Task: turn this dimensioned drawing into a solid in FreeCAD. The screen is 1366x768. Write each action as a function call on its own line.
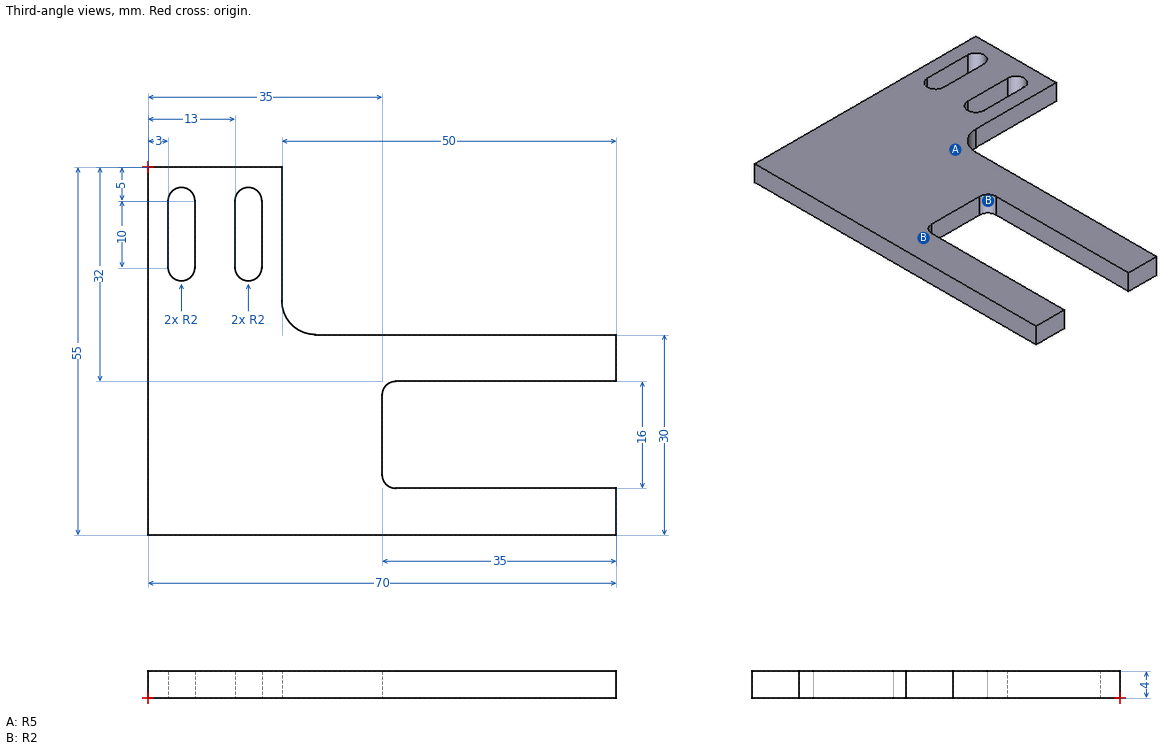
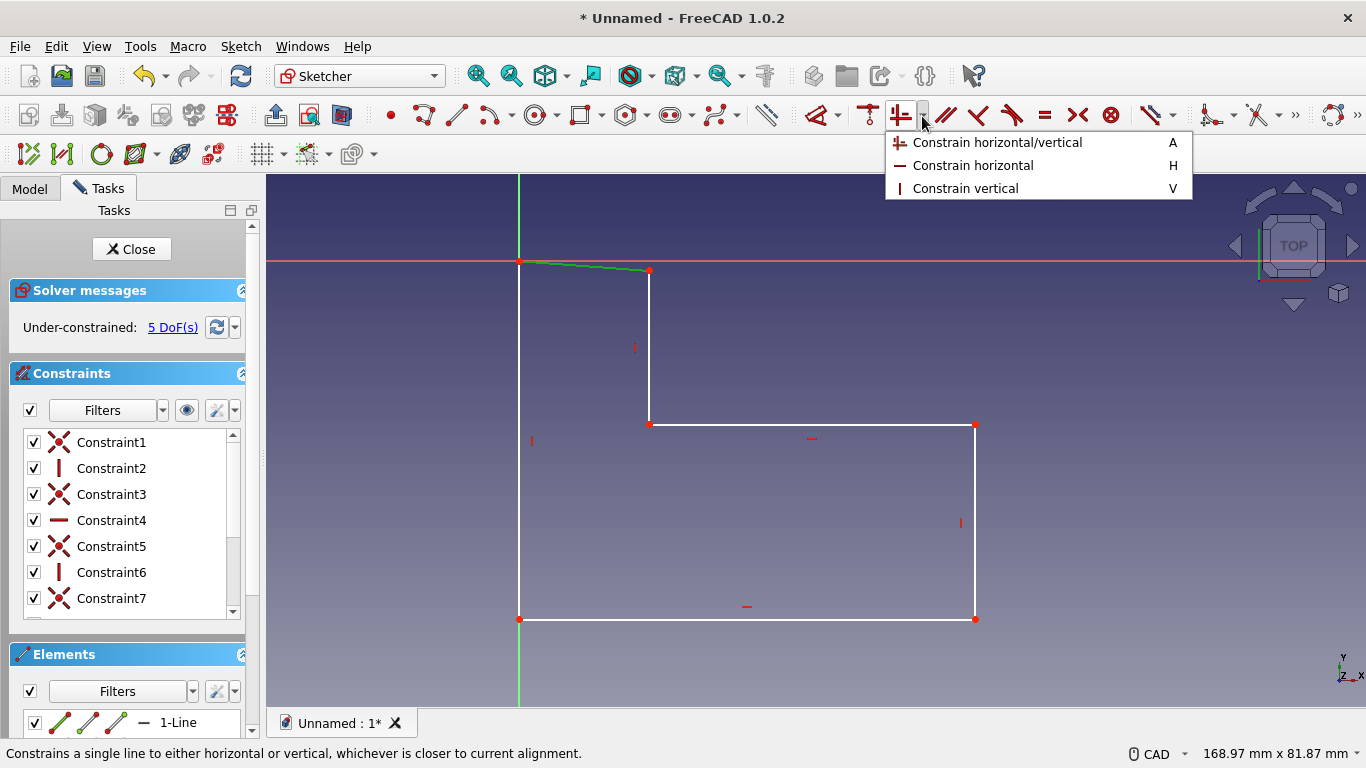
click(1039, 166)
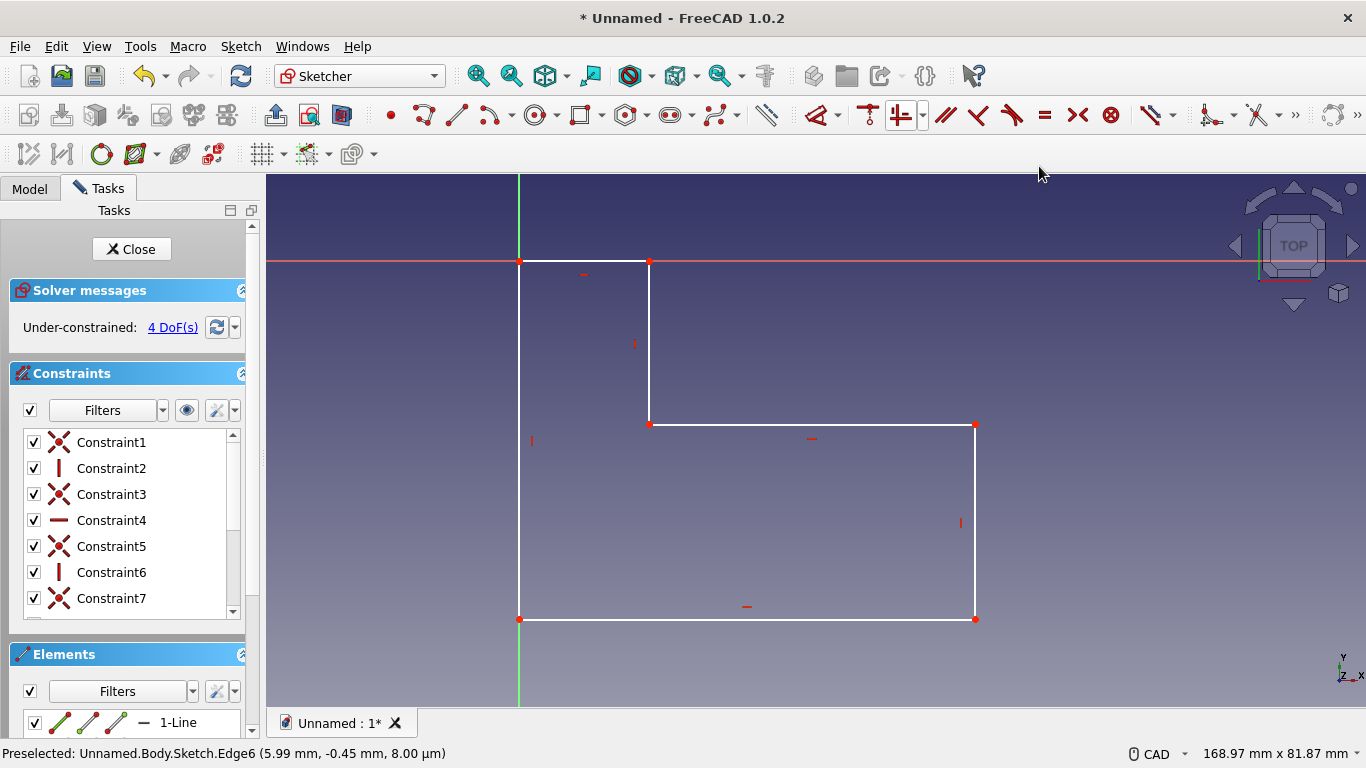
click(816, 116)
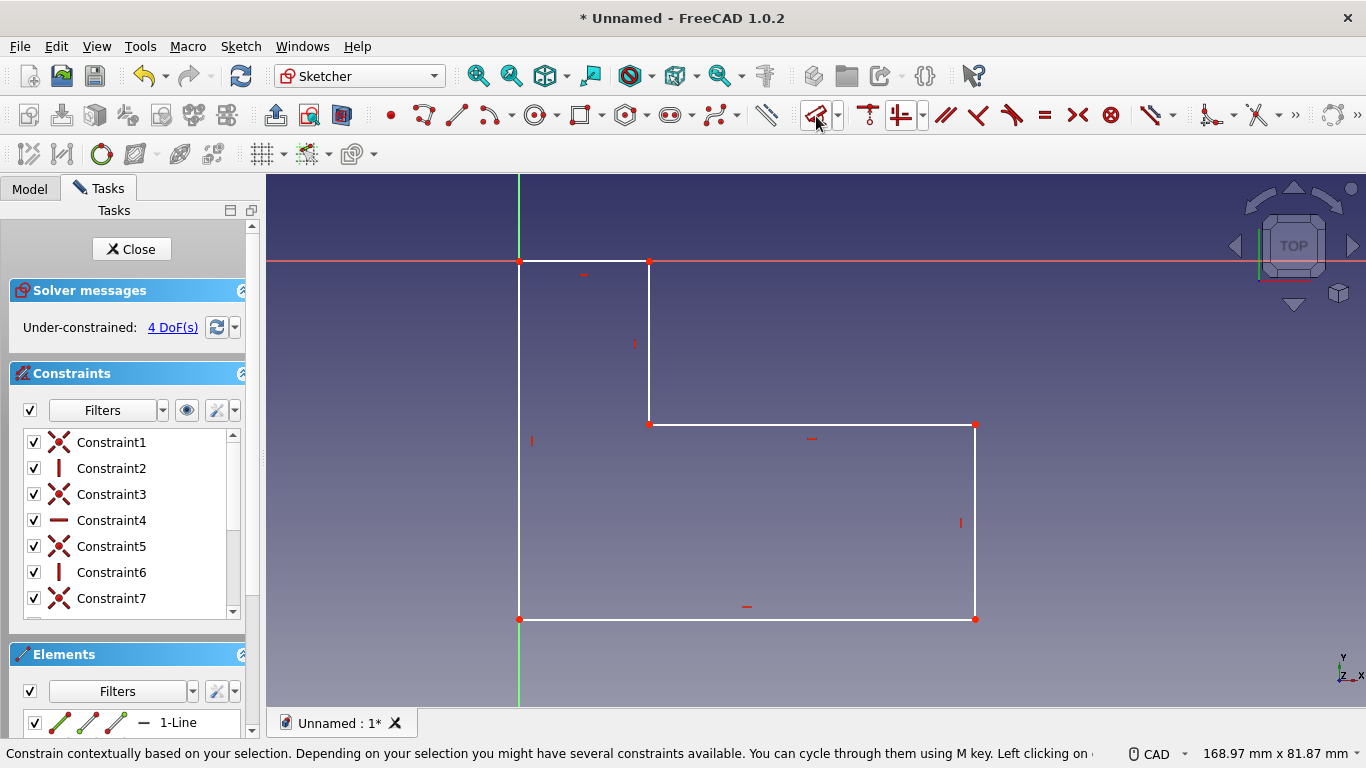
click(519, 369)
click(485, 441)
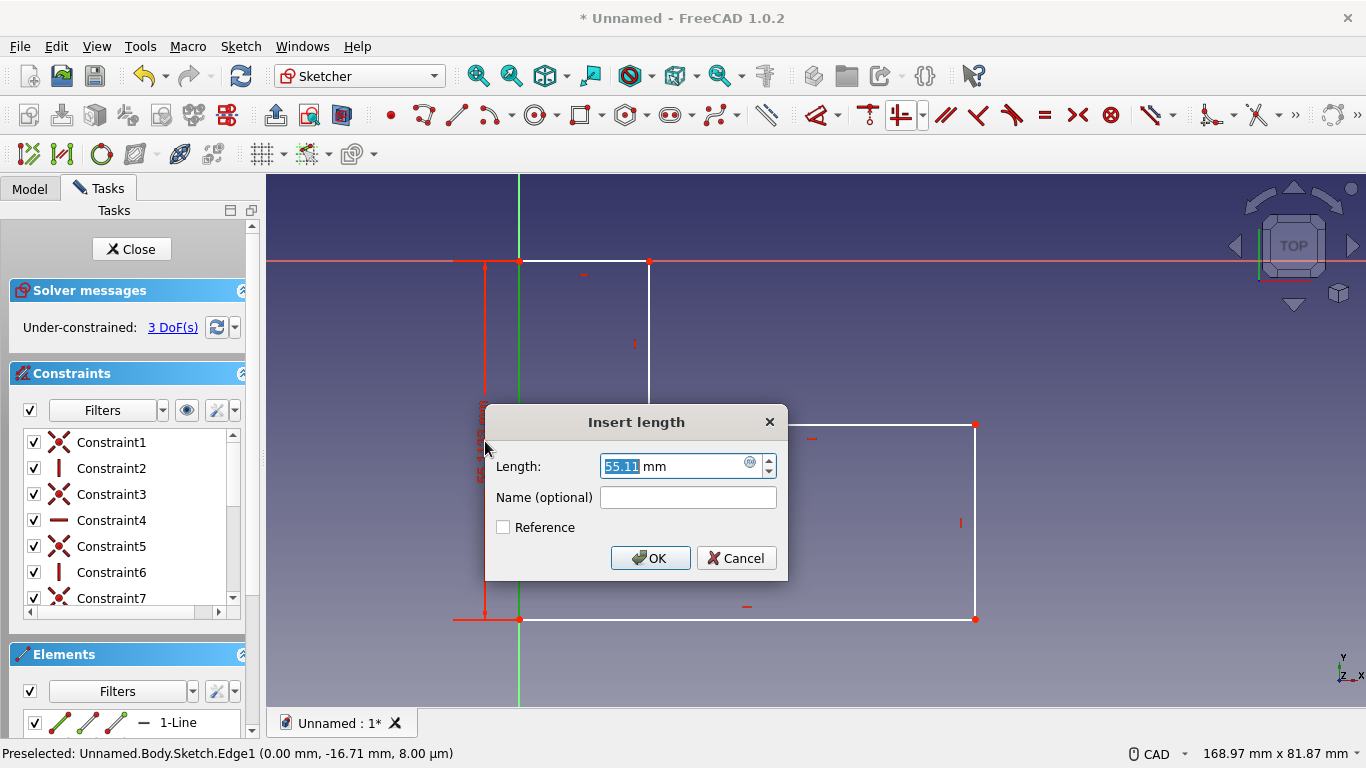
text(55)
key(Return)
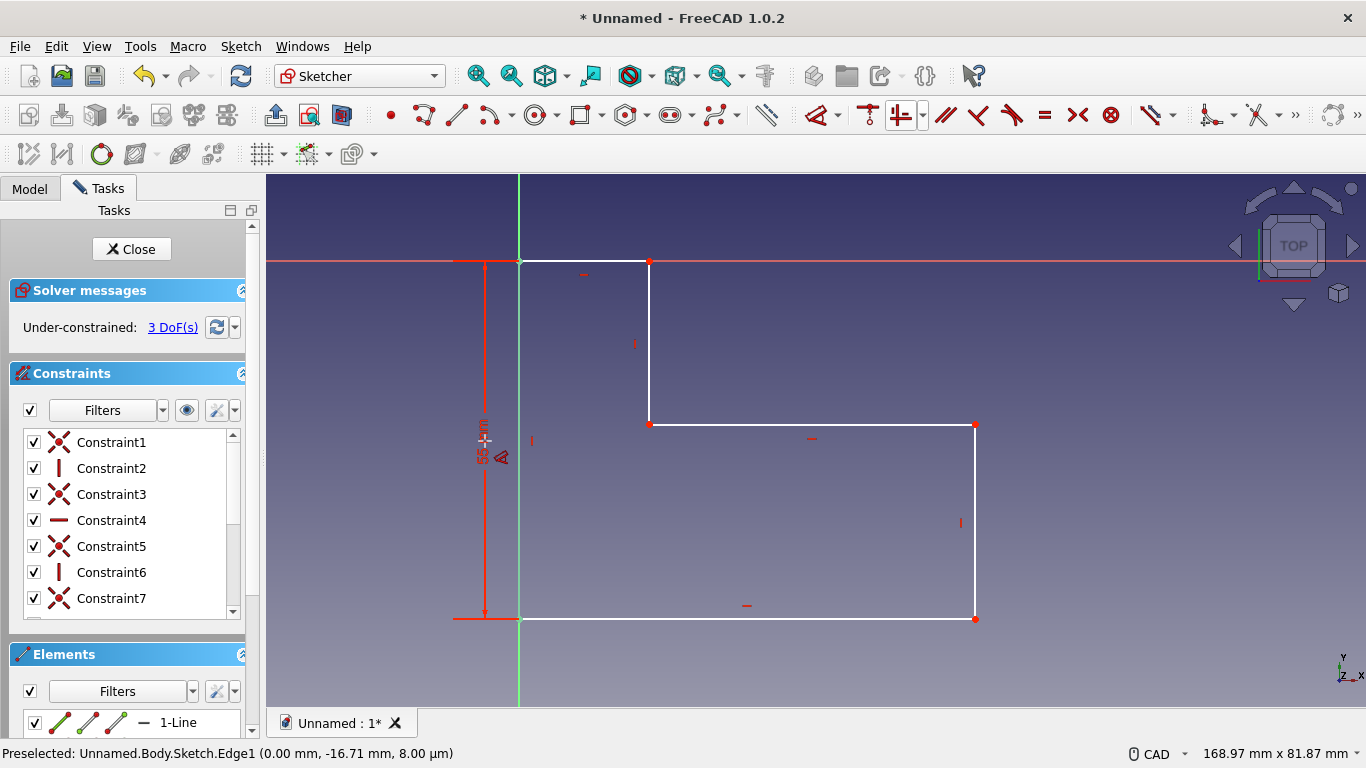
click(656, 619)
click(747, 653)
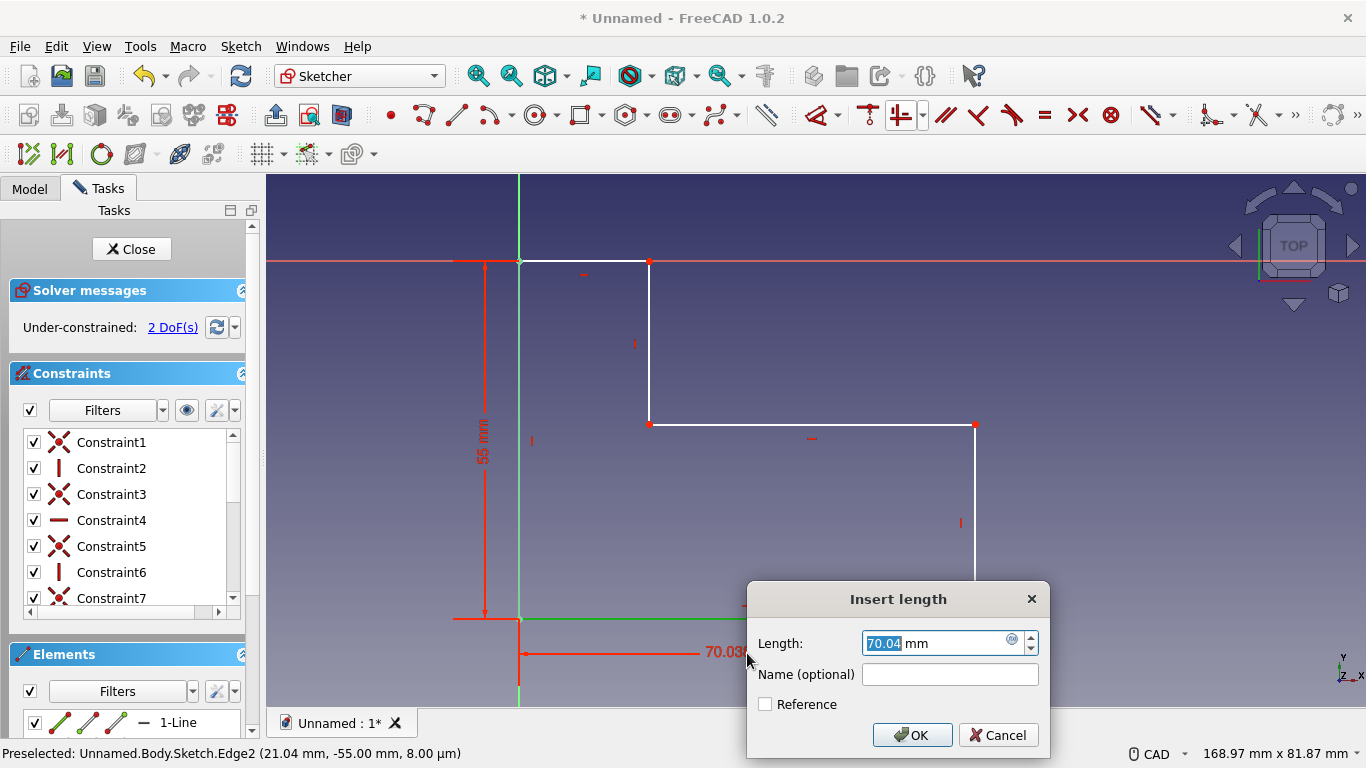
text(70)
key(Return)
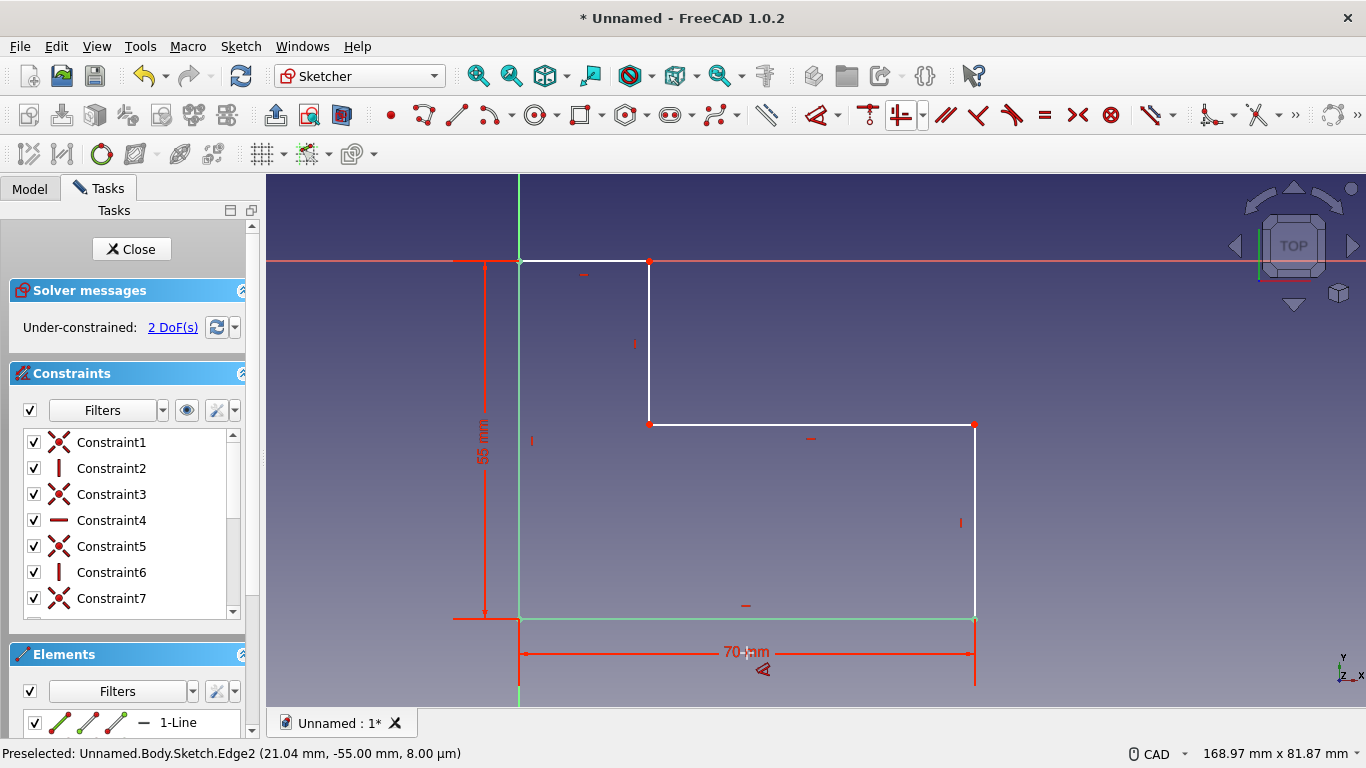
click(975, 561)
click(1009, 522)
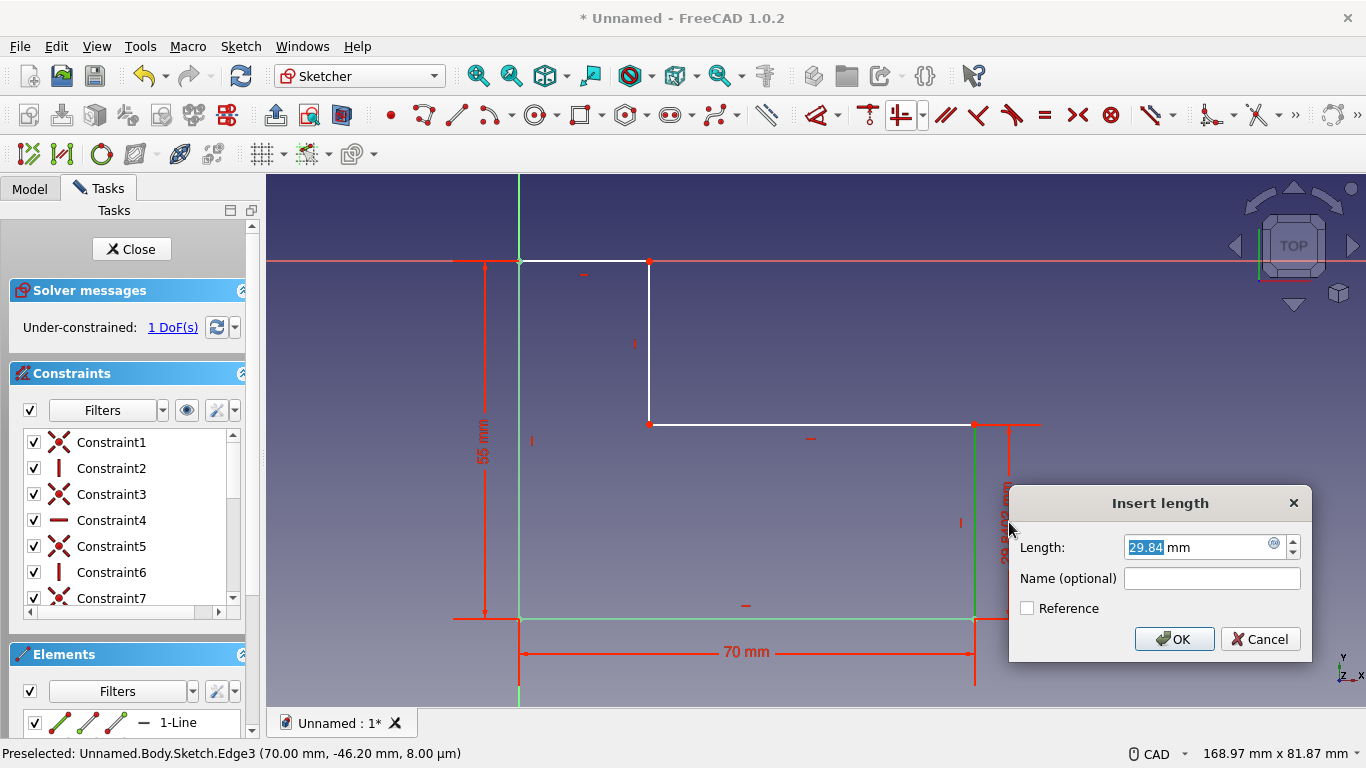
text(30)
key(Return)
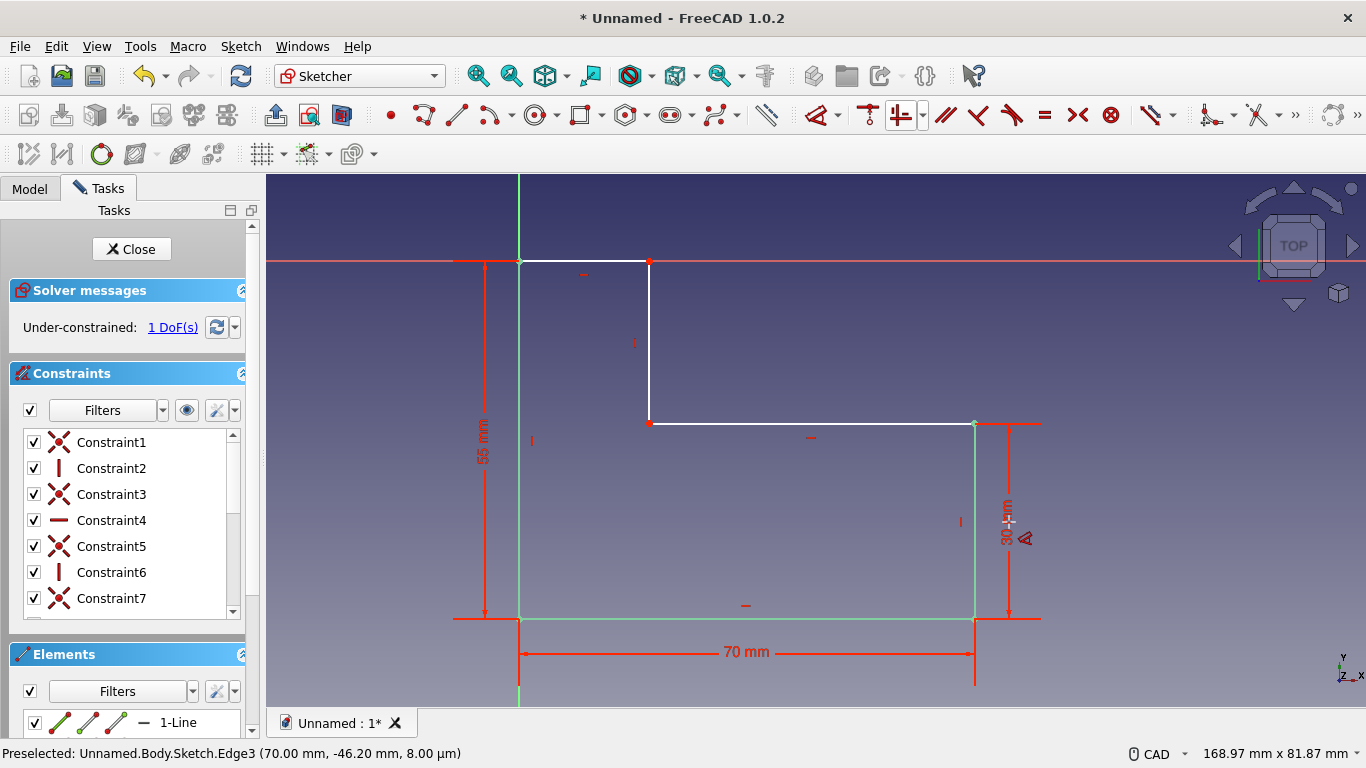
click(877, 424)
click(812, 390)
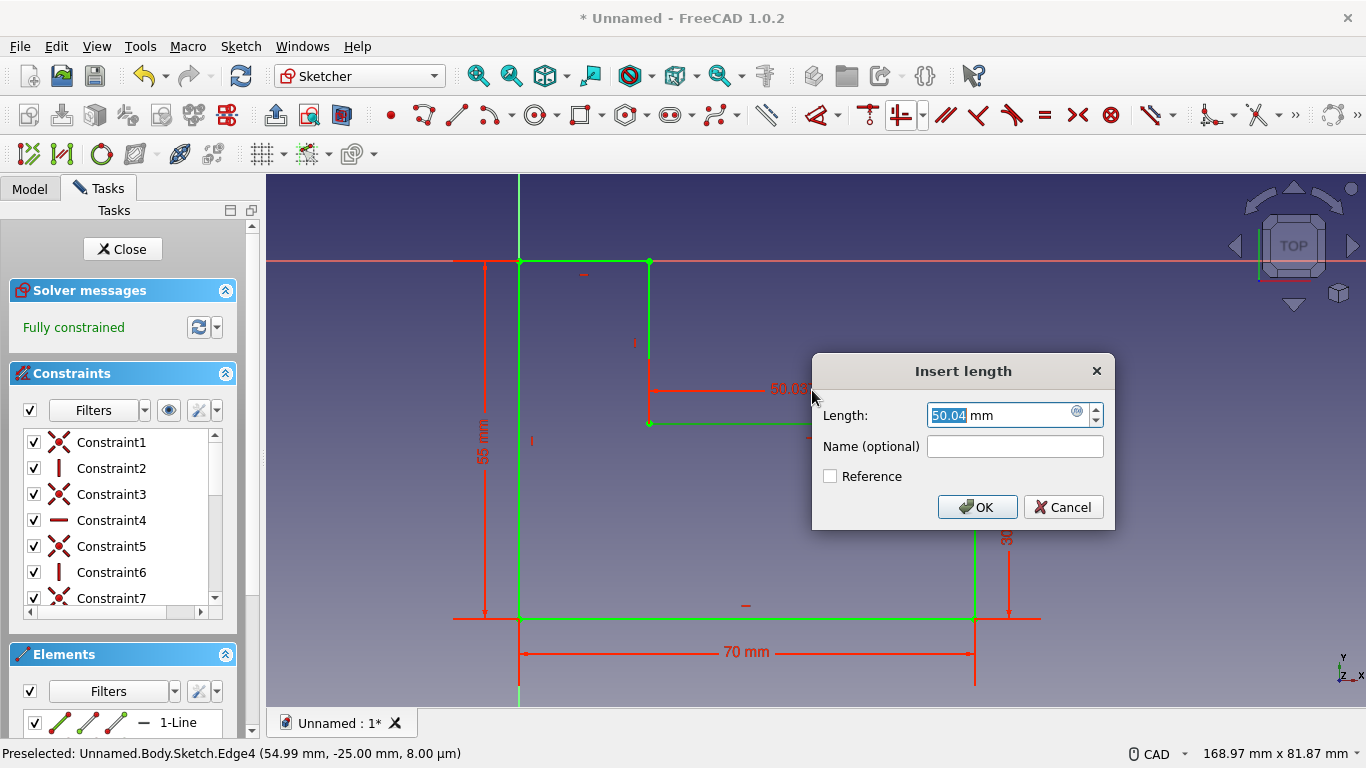
text(50)
key(Return)
key(Escape)